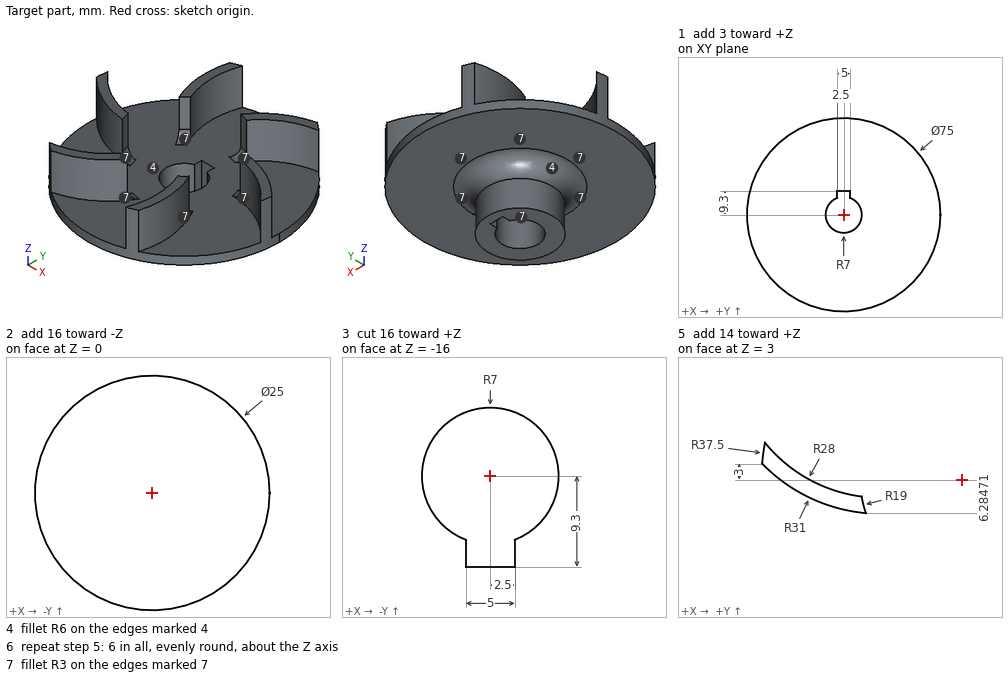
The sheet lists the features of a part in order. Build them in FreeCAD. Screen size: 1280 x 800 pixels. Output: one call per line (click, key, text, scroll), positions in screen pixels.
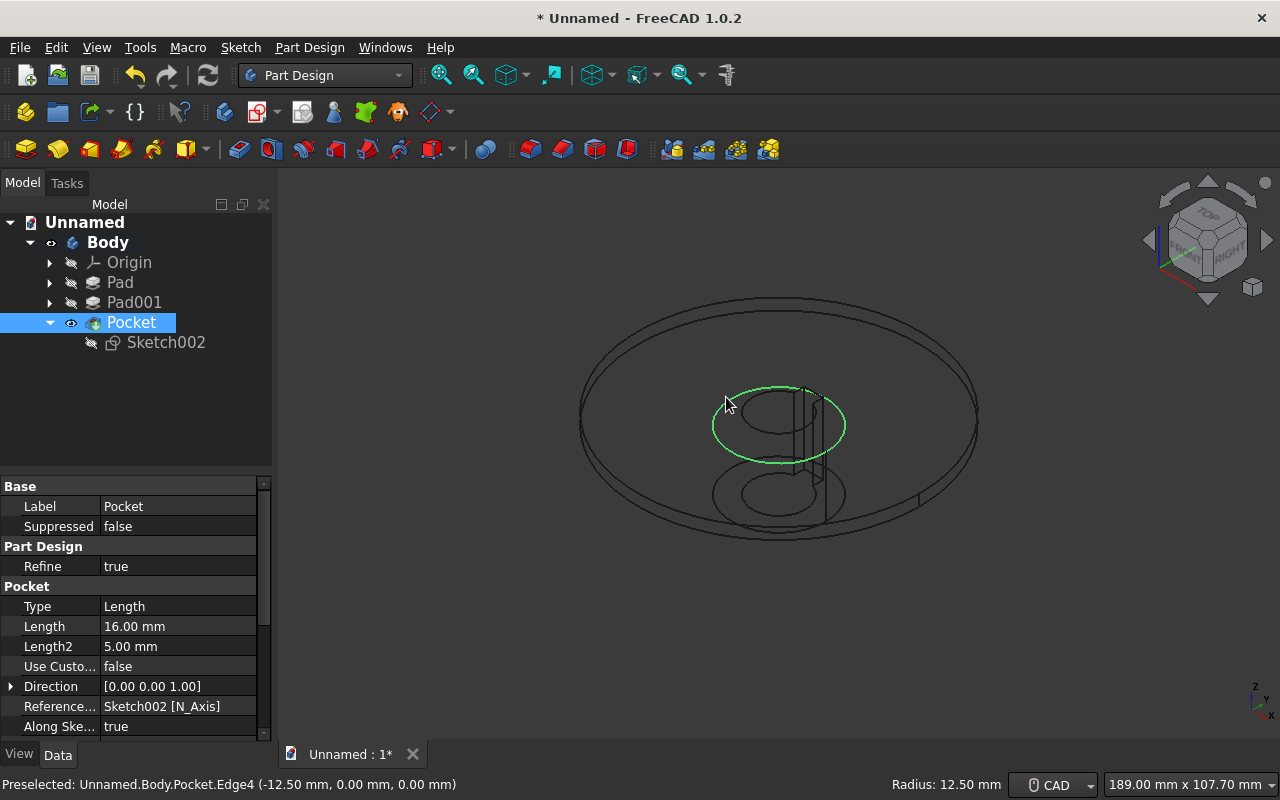
key(v)
key(1)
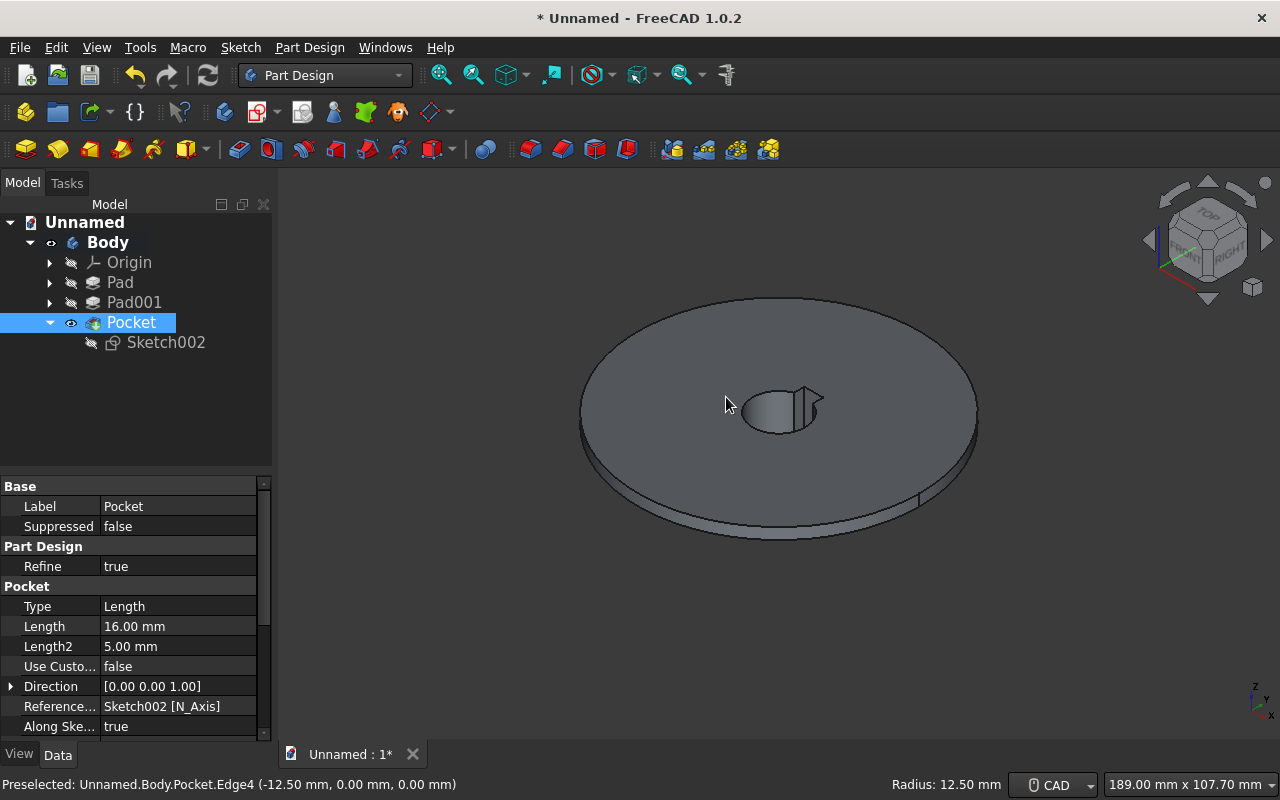
click(532, 150)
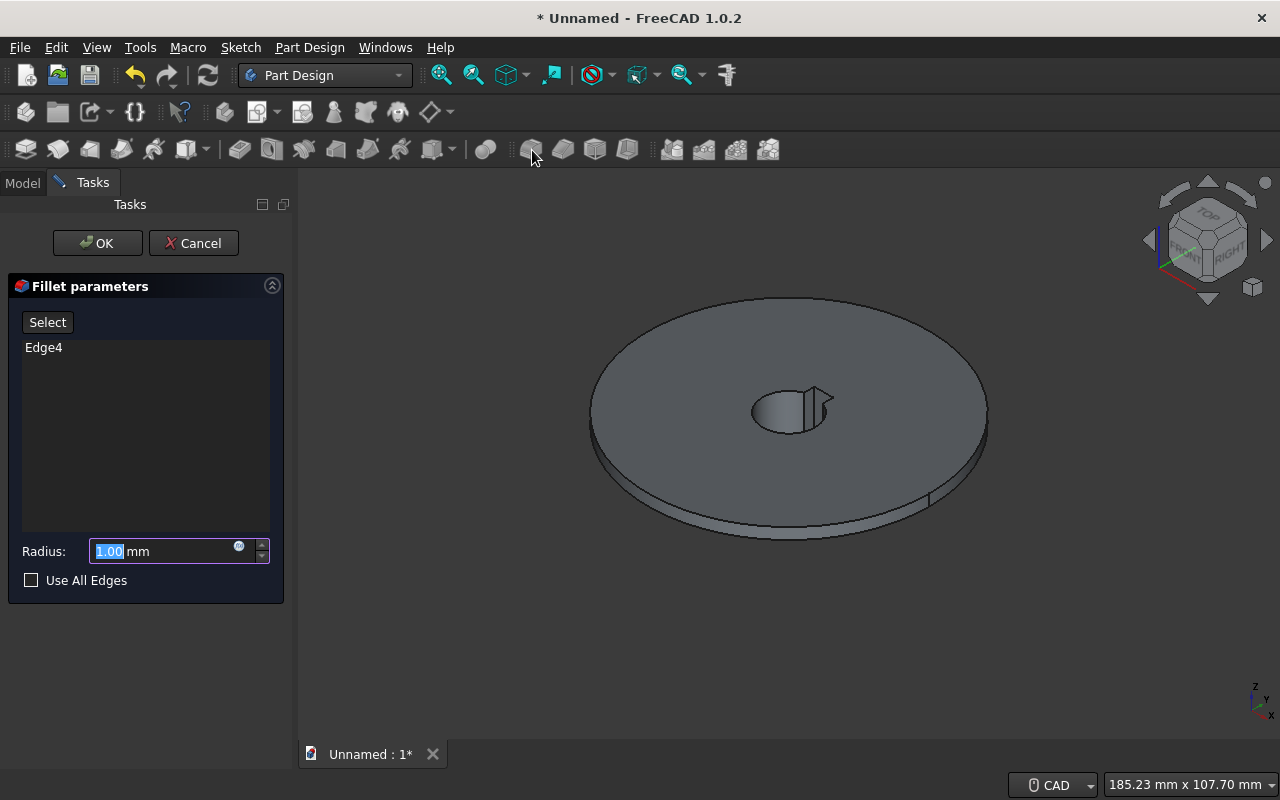
text(6)
key(Tab)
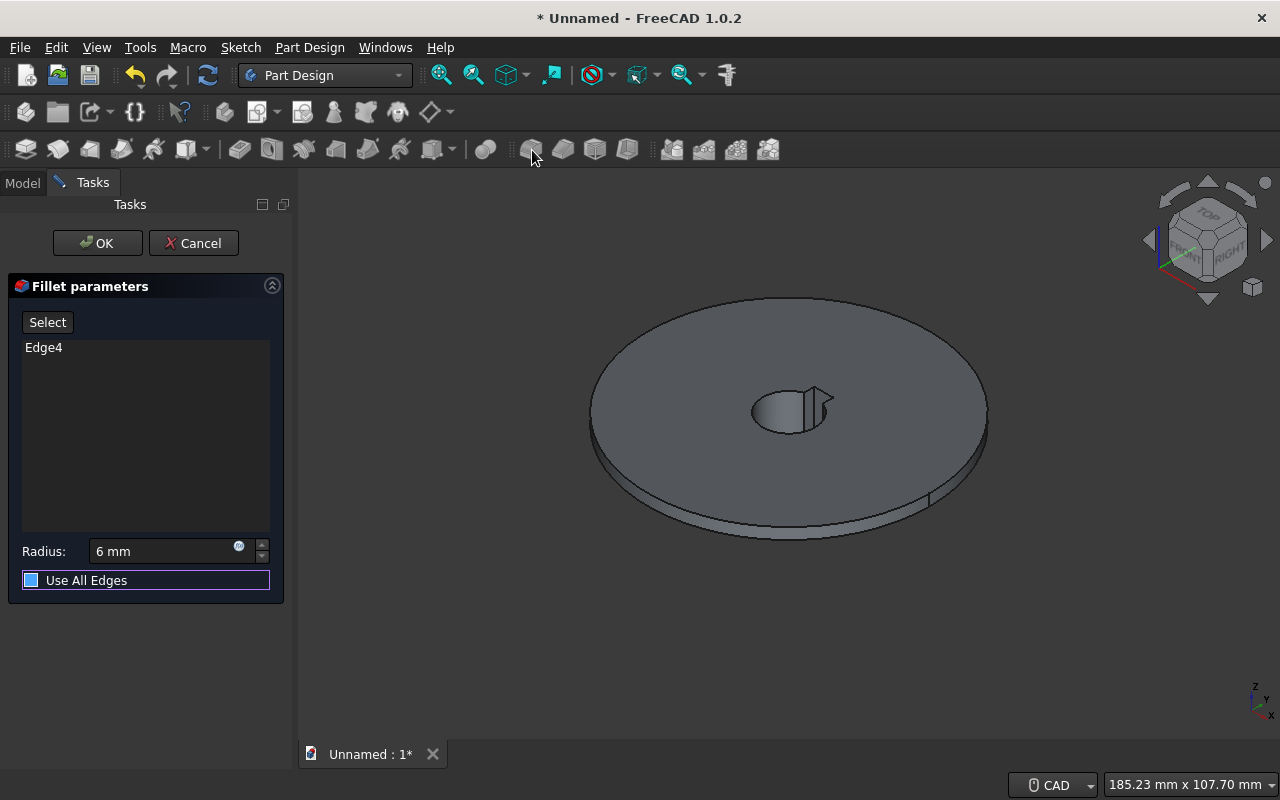
click(98, 243)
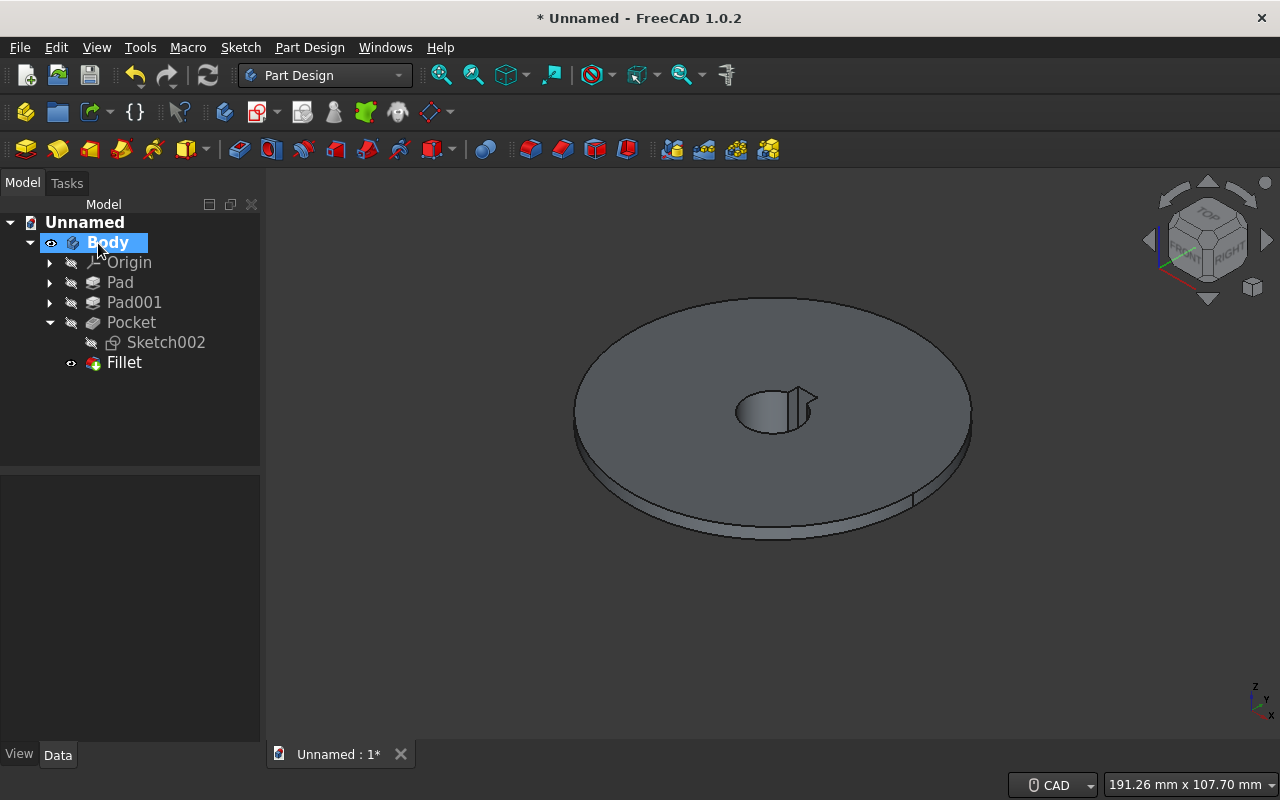
click(693, 365)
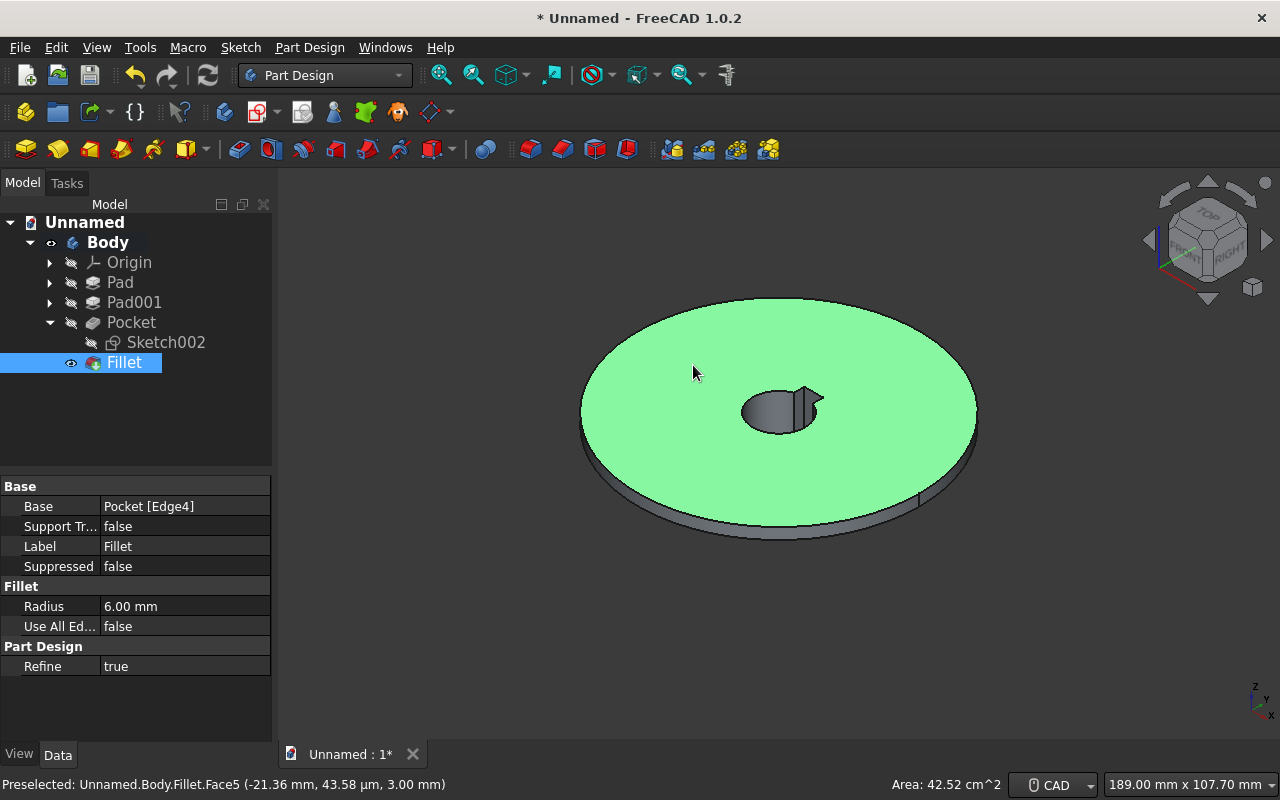
click(258, 112)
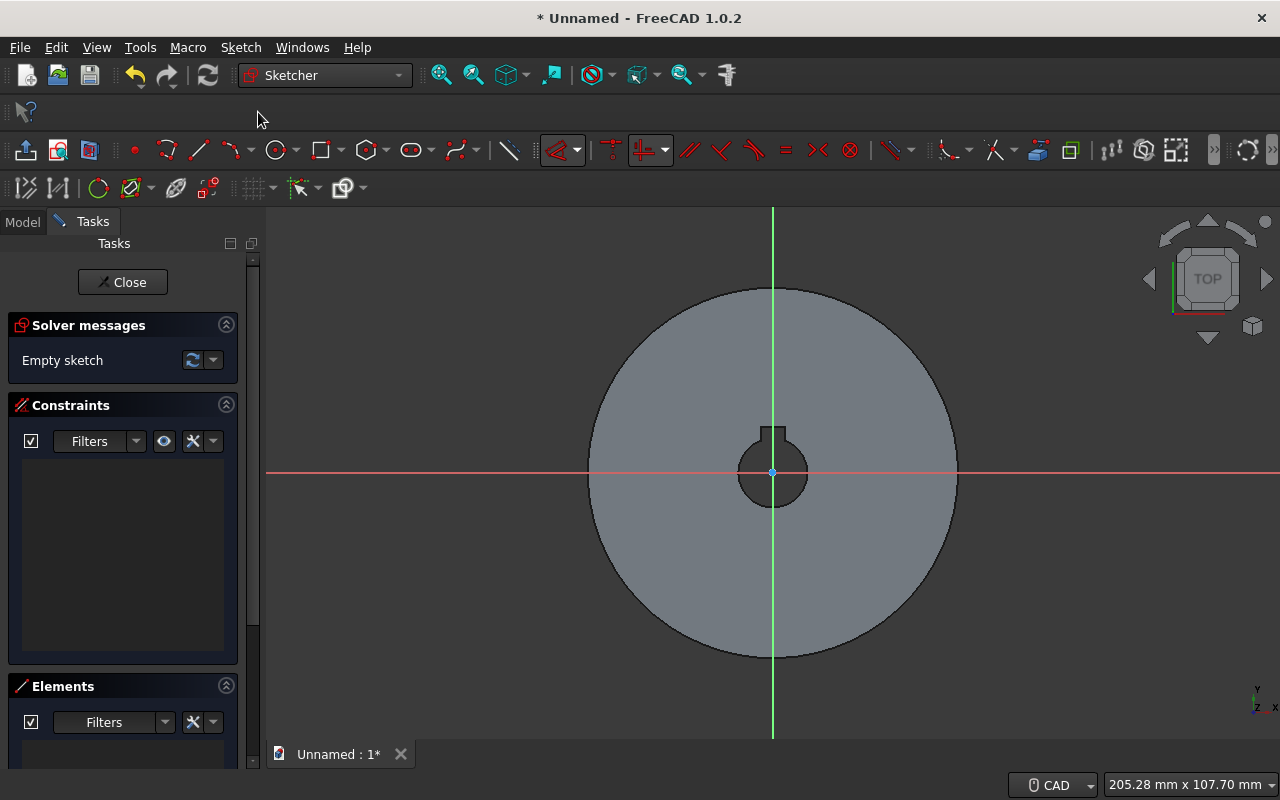
scroll(670, 471, up, 6)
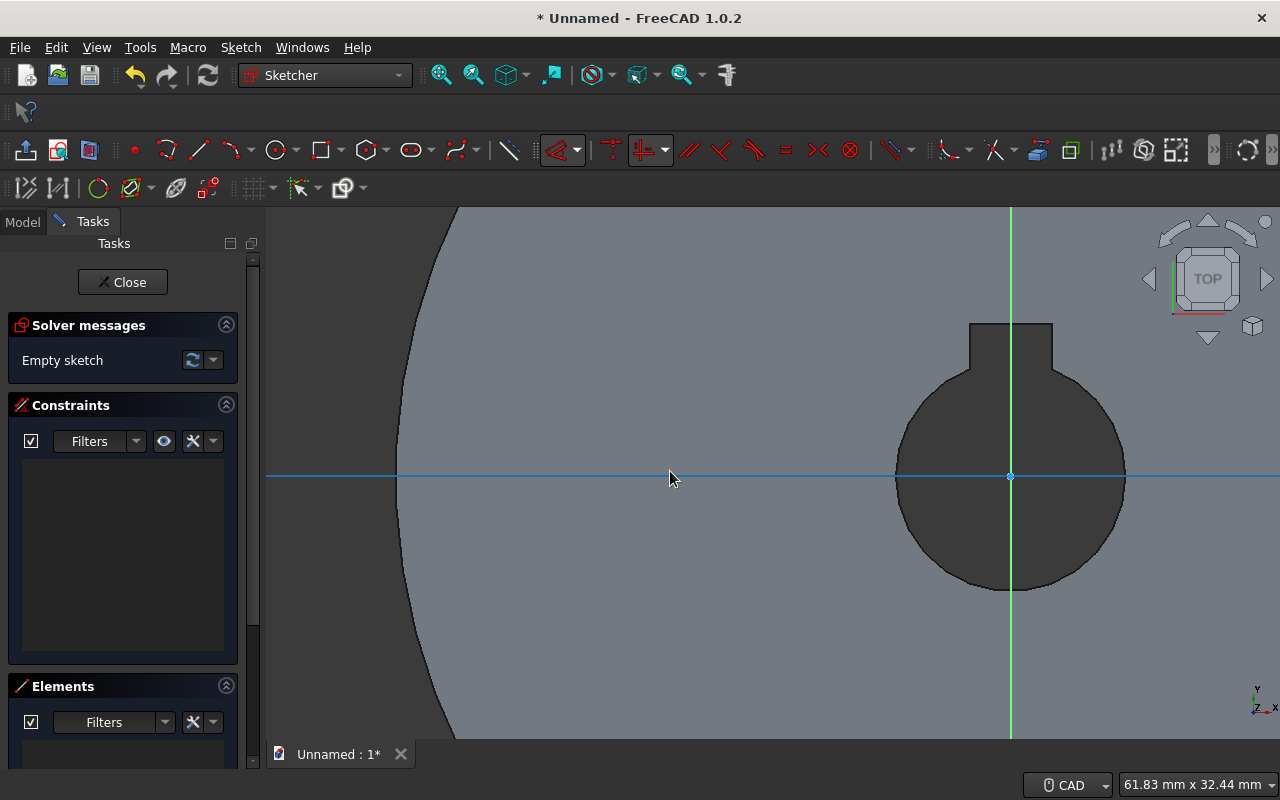
click(232, 150)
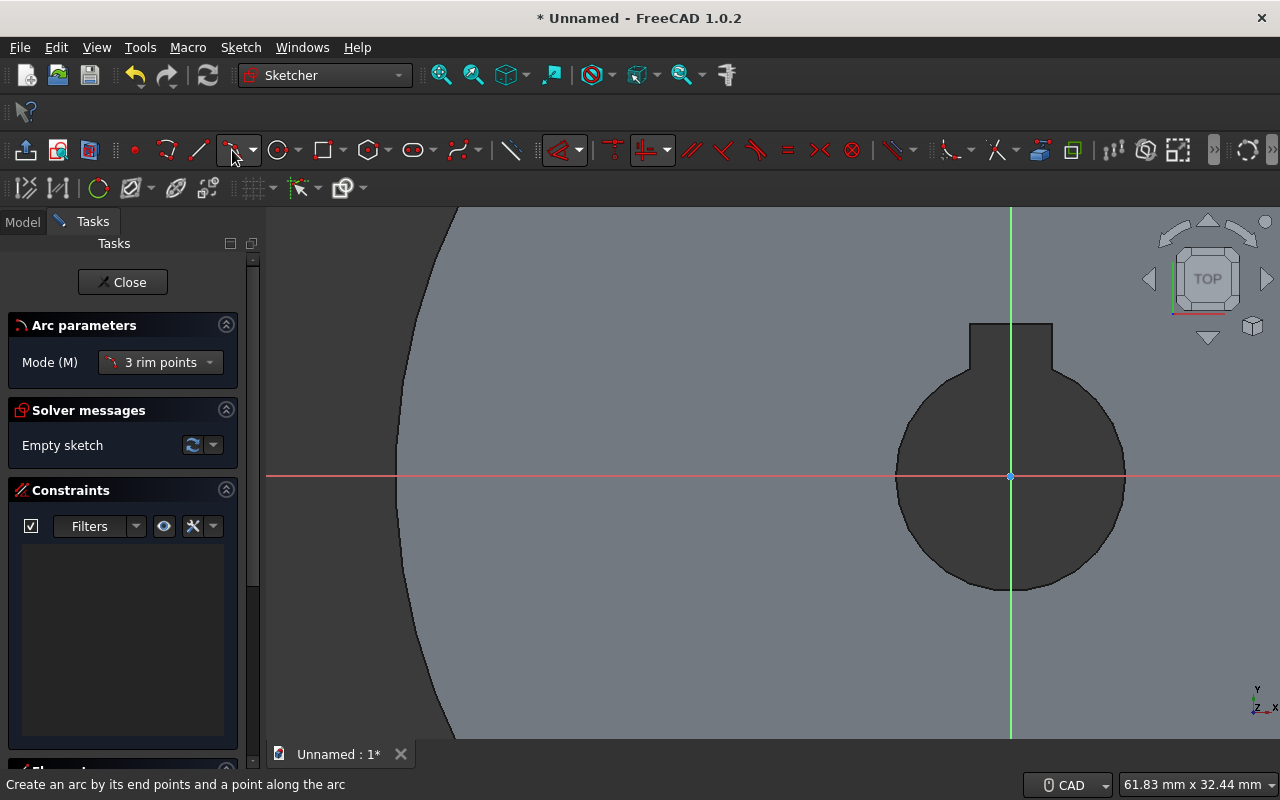
click(717, 580)
click(703, 529)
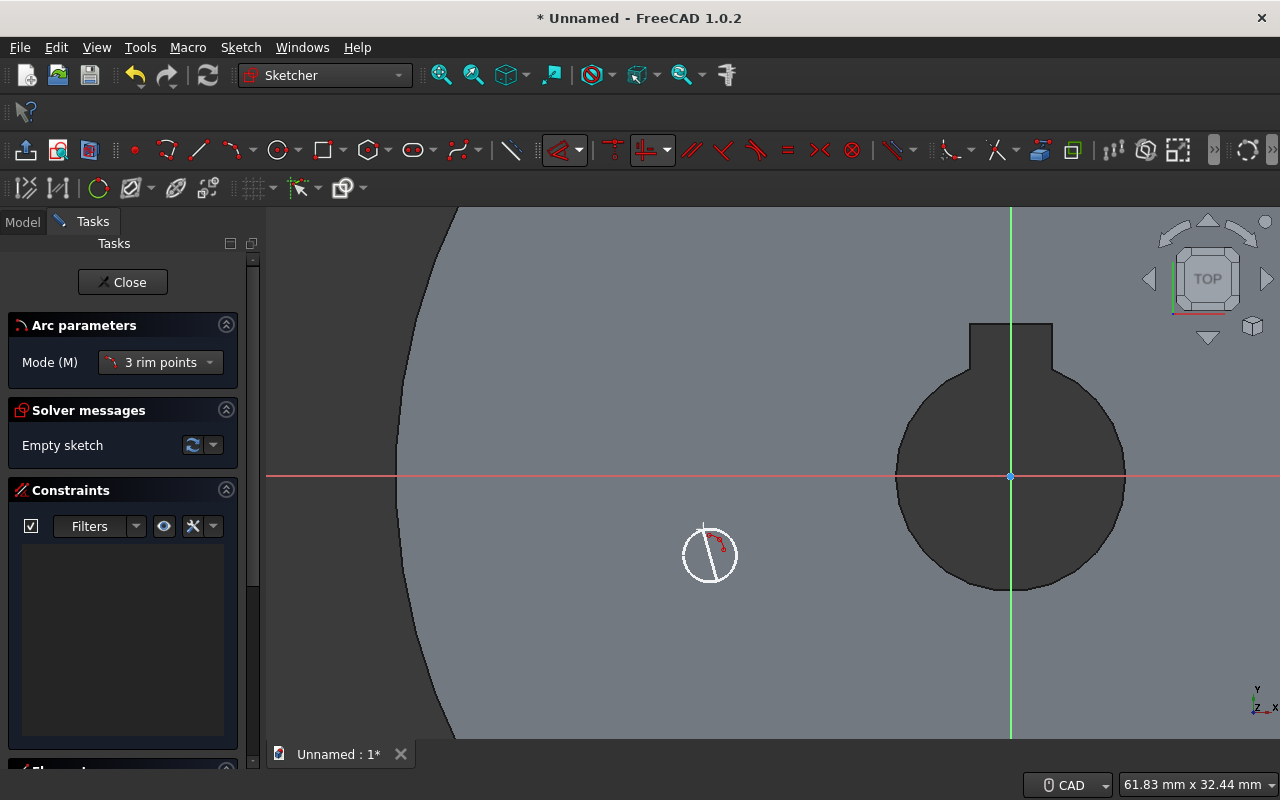
scroll(709, 554, up, 14)